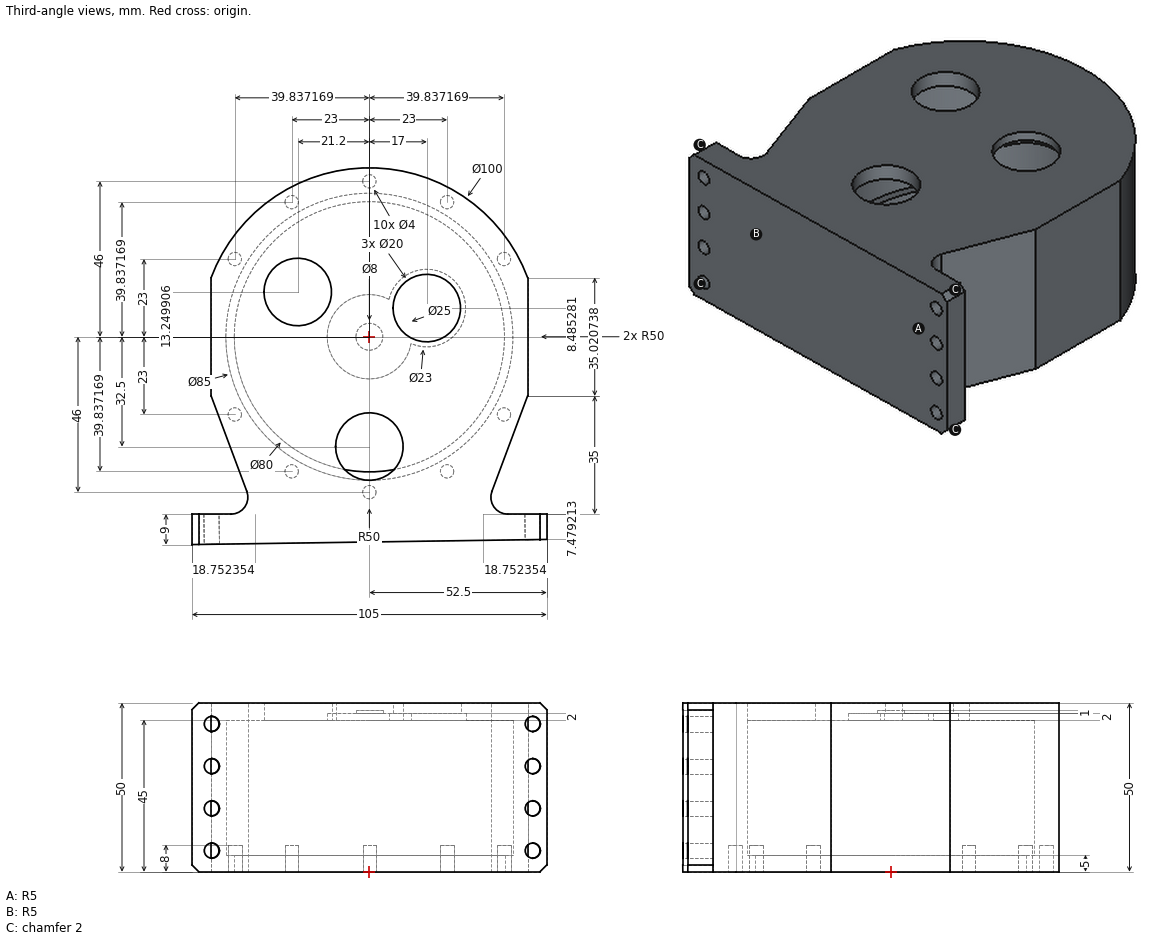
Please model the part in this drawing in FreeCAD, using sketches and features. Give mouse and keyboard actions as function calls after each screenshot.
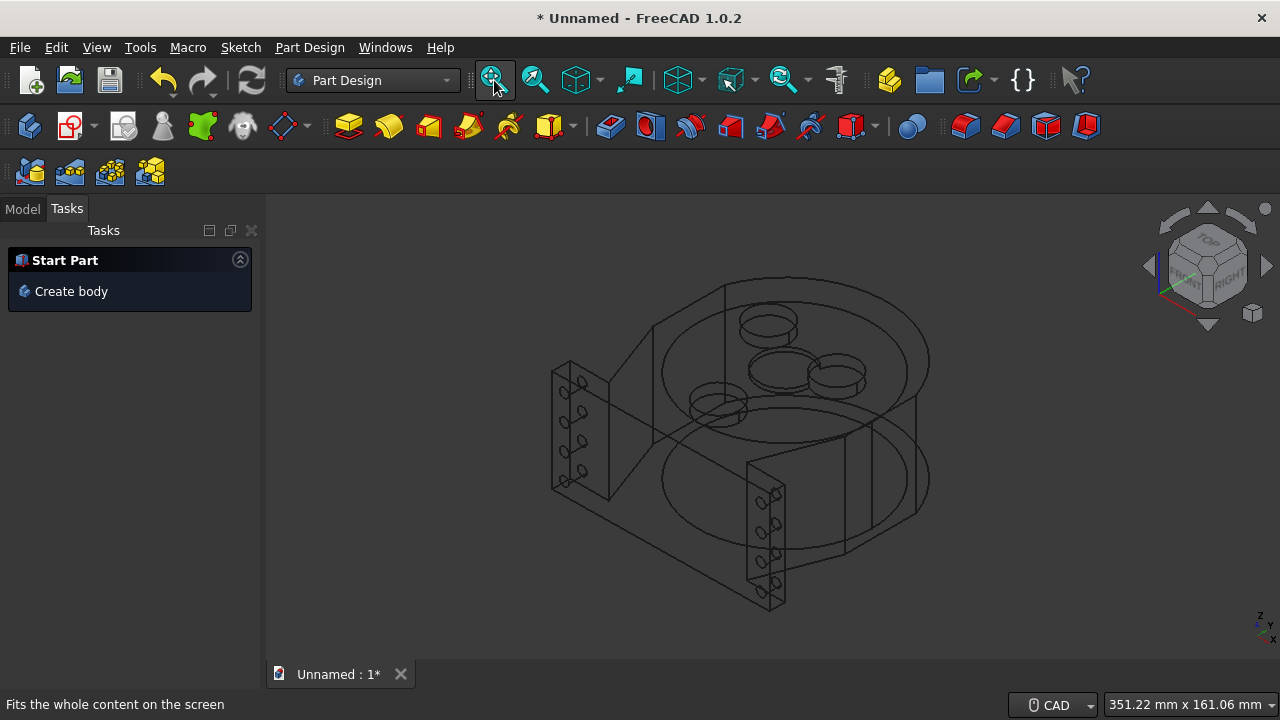
click(747, 520)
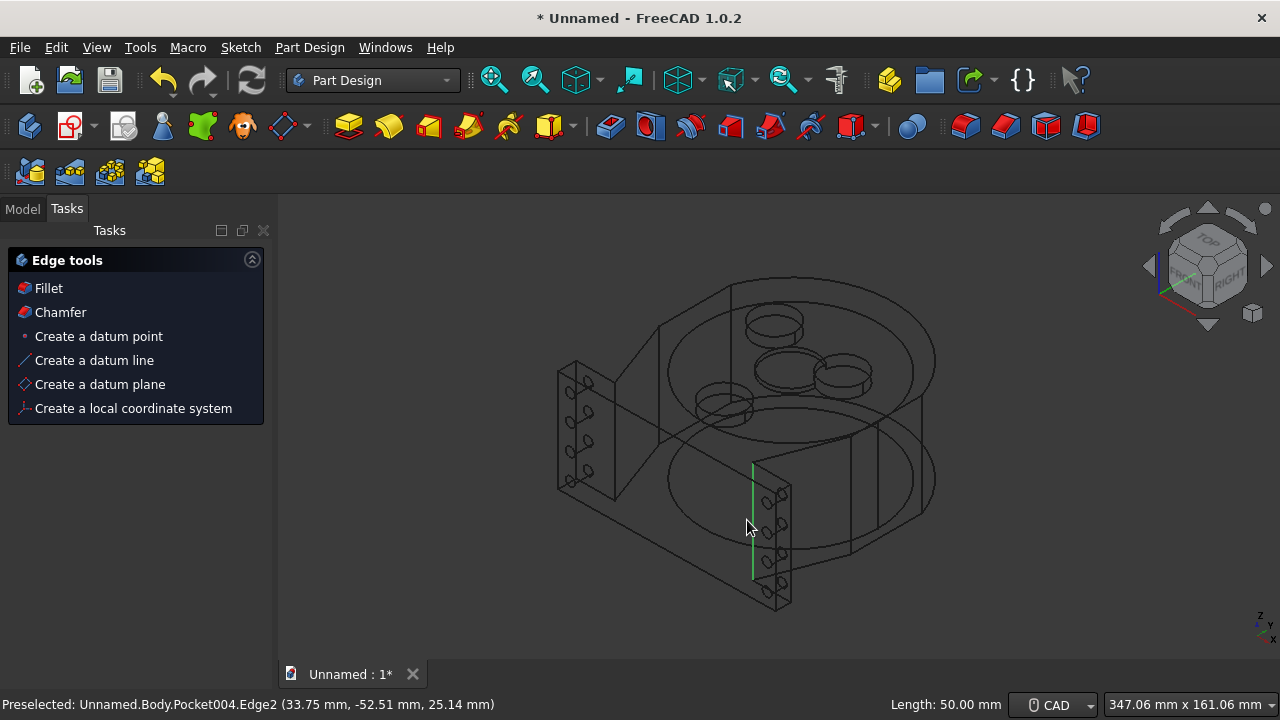
key(v)
key(1)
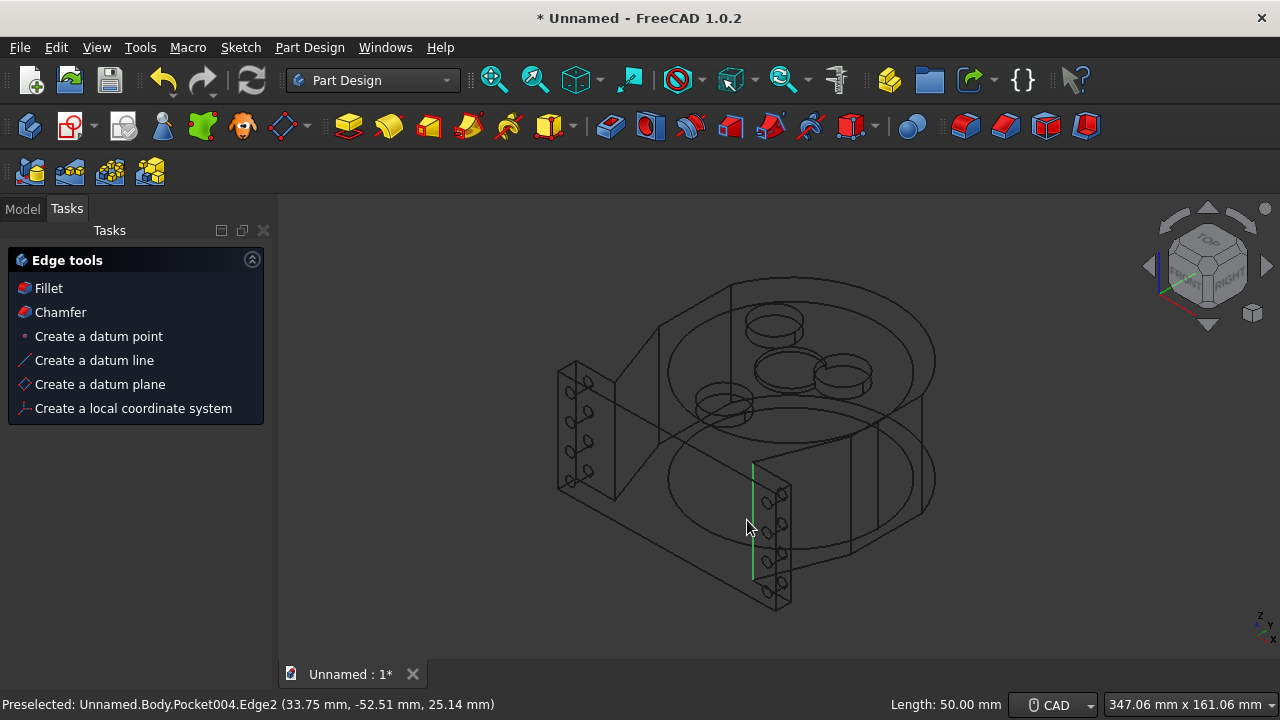
click(966, 126)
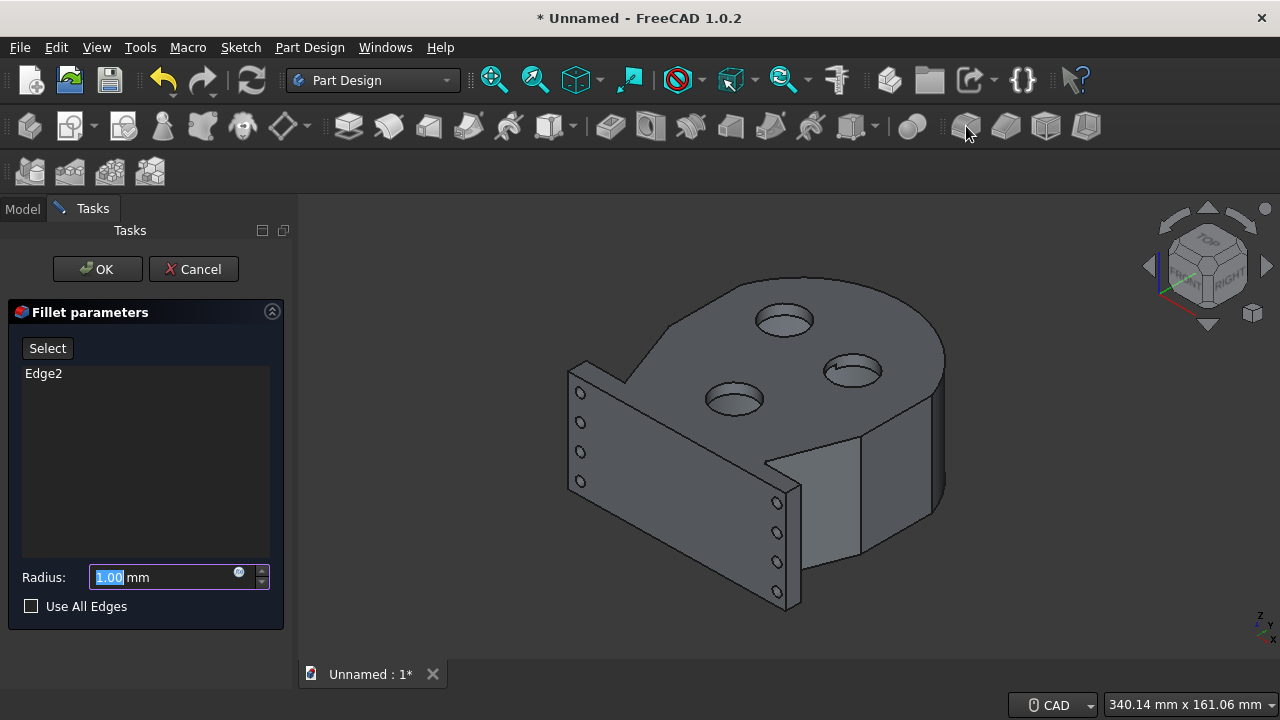
text(5)
key(Tab)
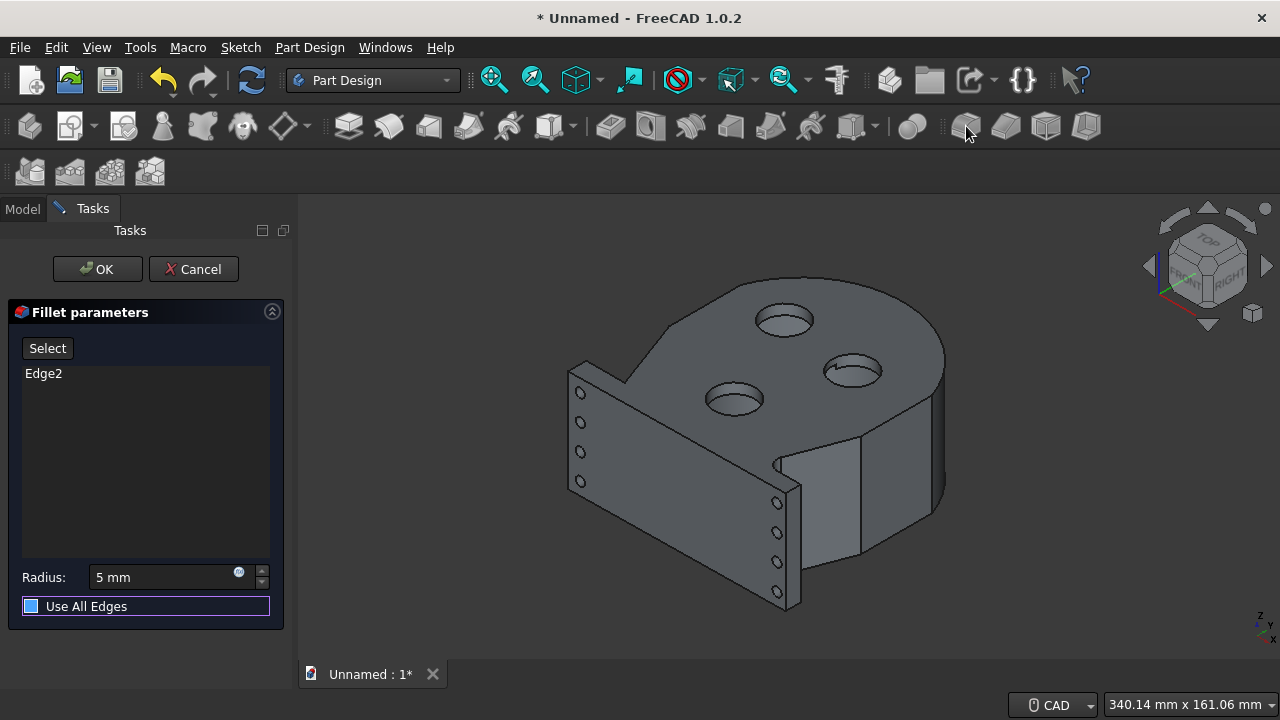
click(98, 269)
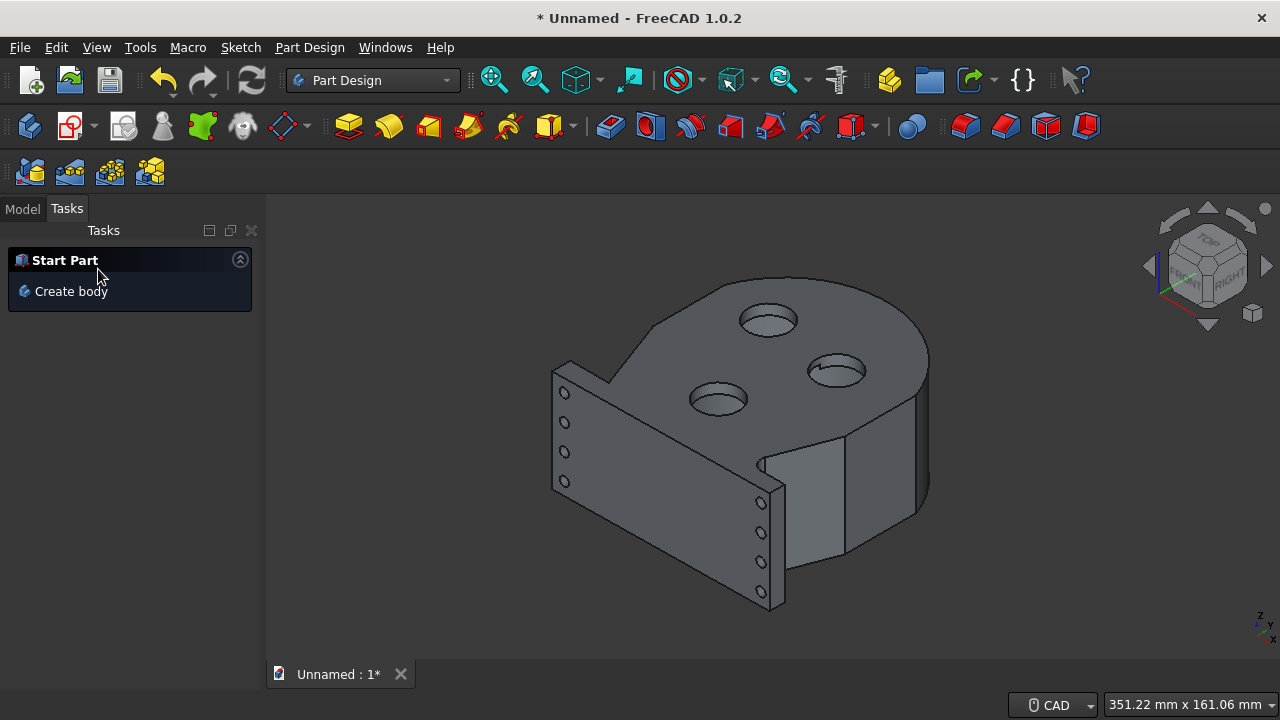
key(2)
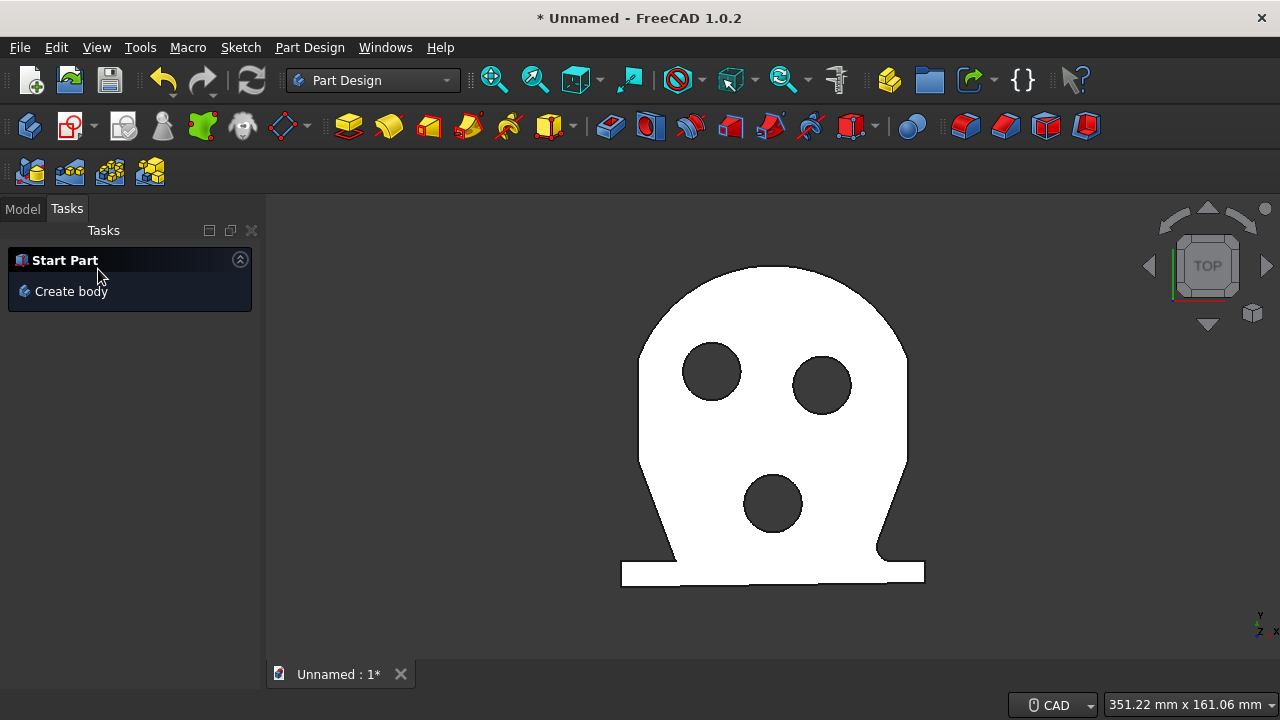
key(0)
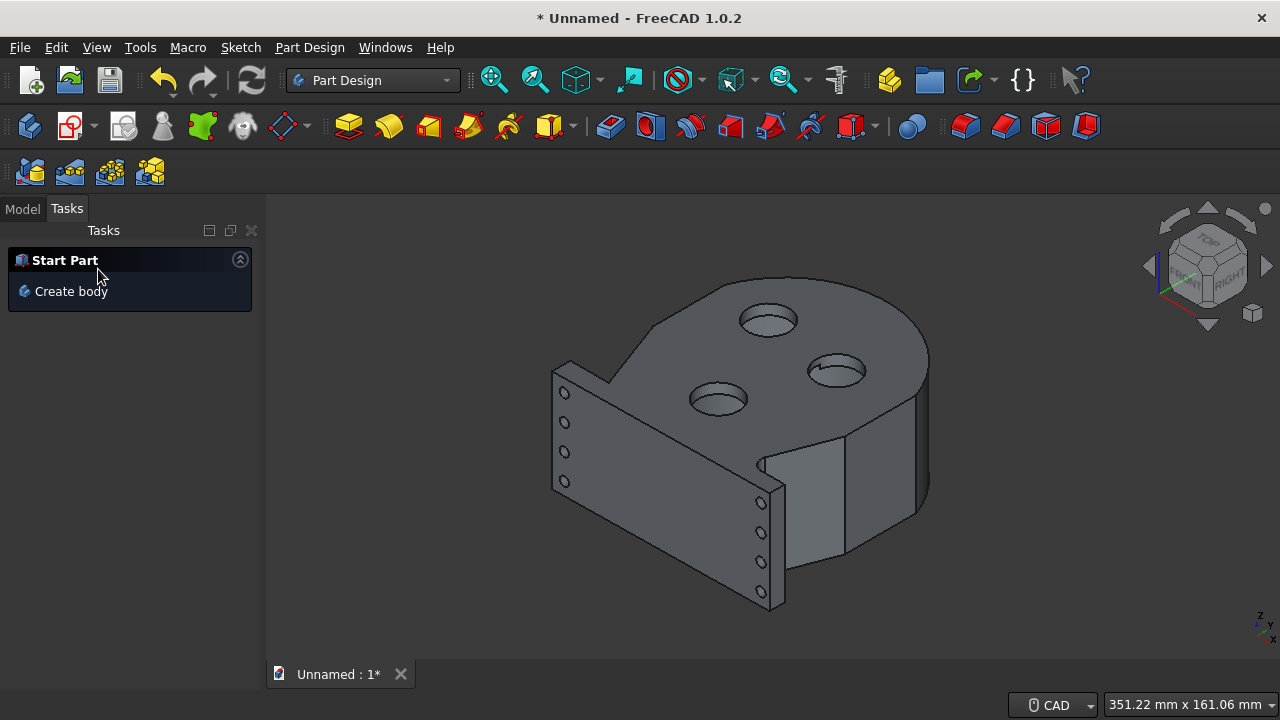
key(1)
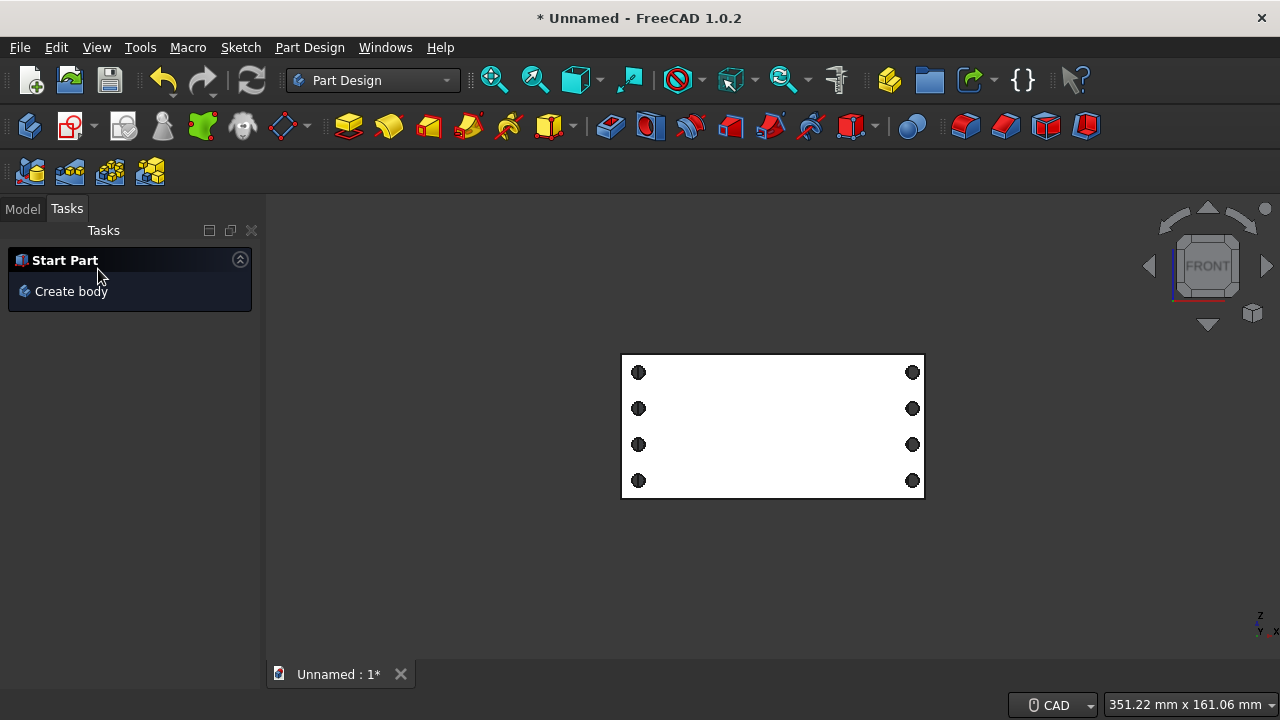
click(496, 80)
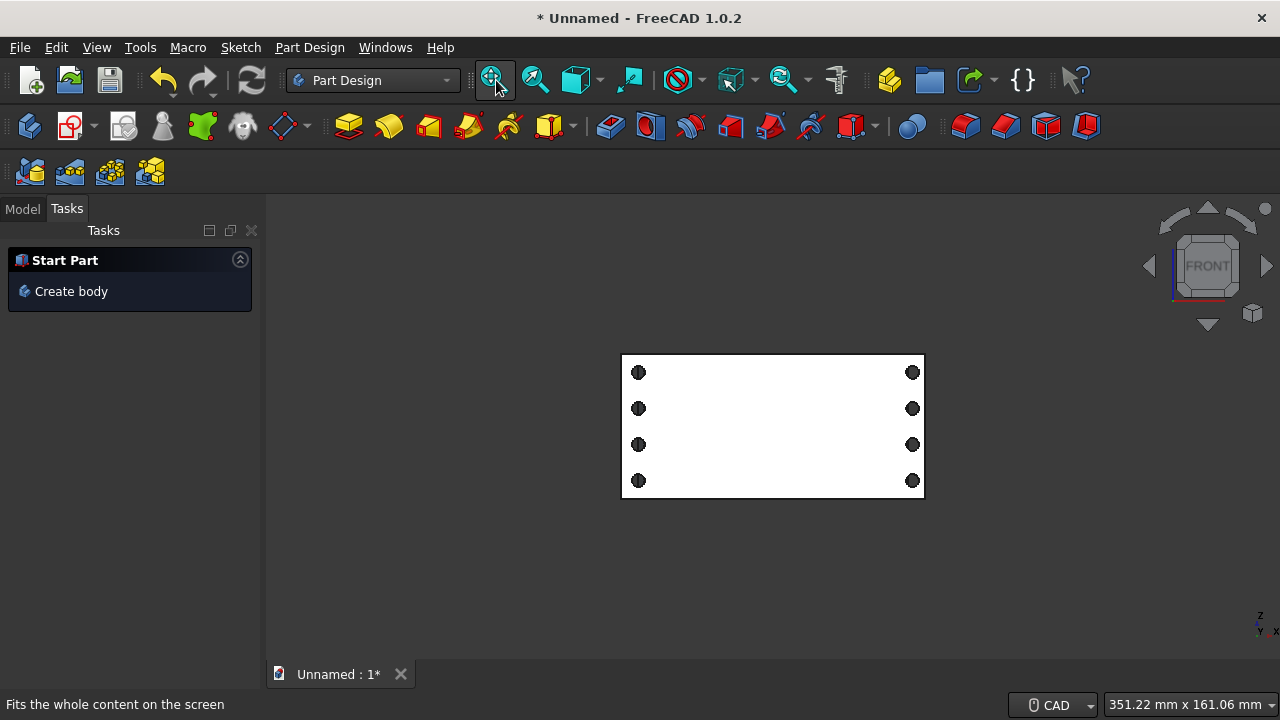
key(3)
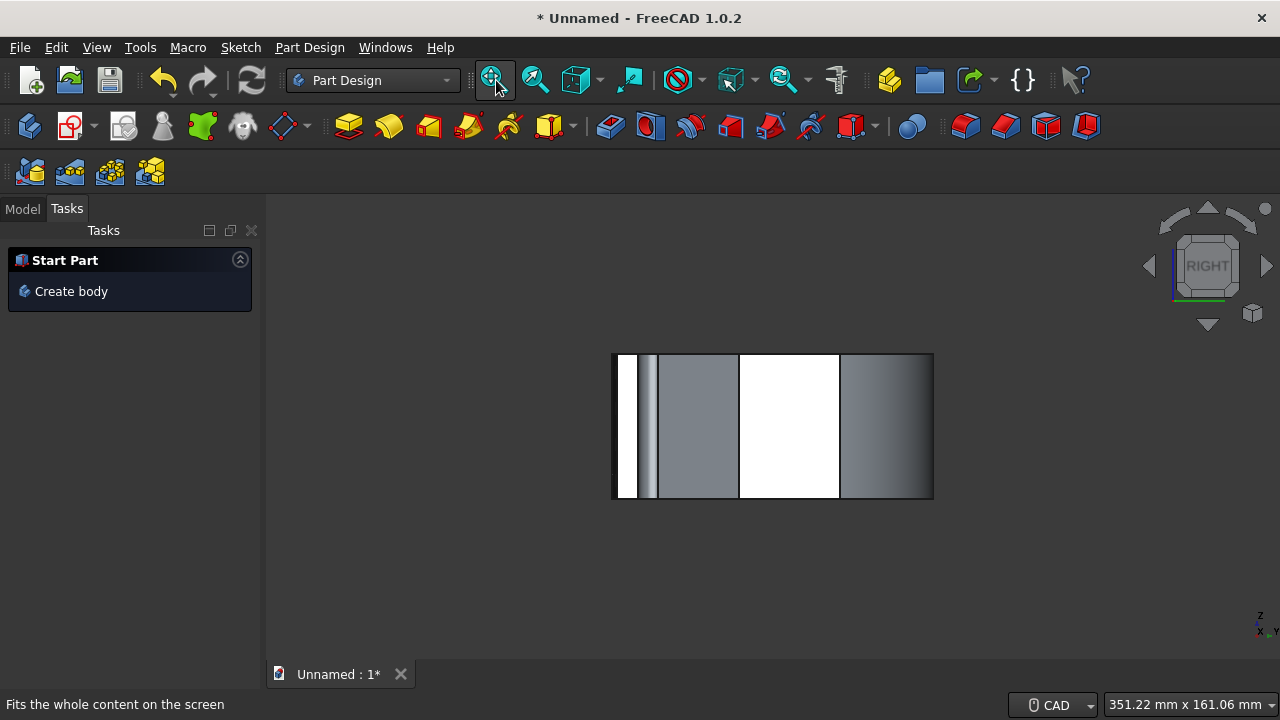
click(496, 80)